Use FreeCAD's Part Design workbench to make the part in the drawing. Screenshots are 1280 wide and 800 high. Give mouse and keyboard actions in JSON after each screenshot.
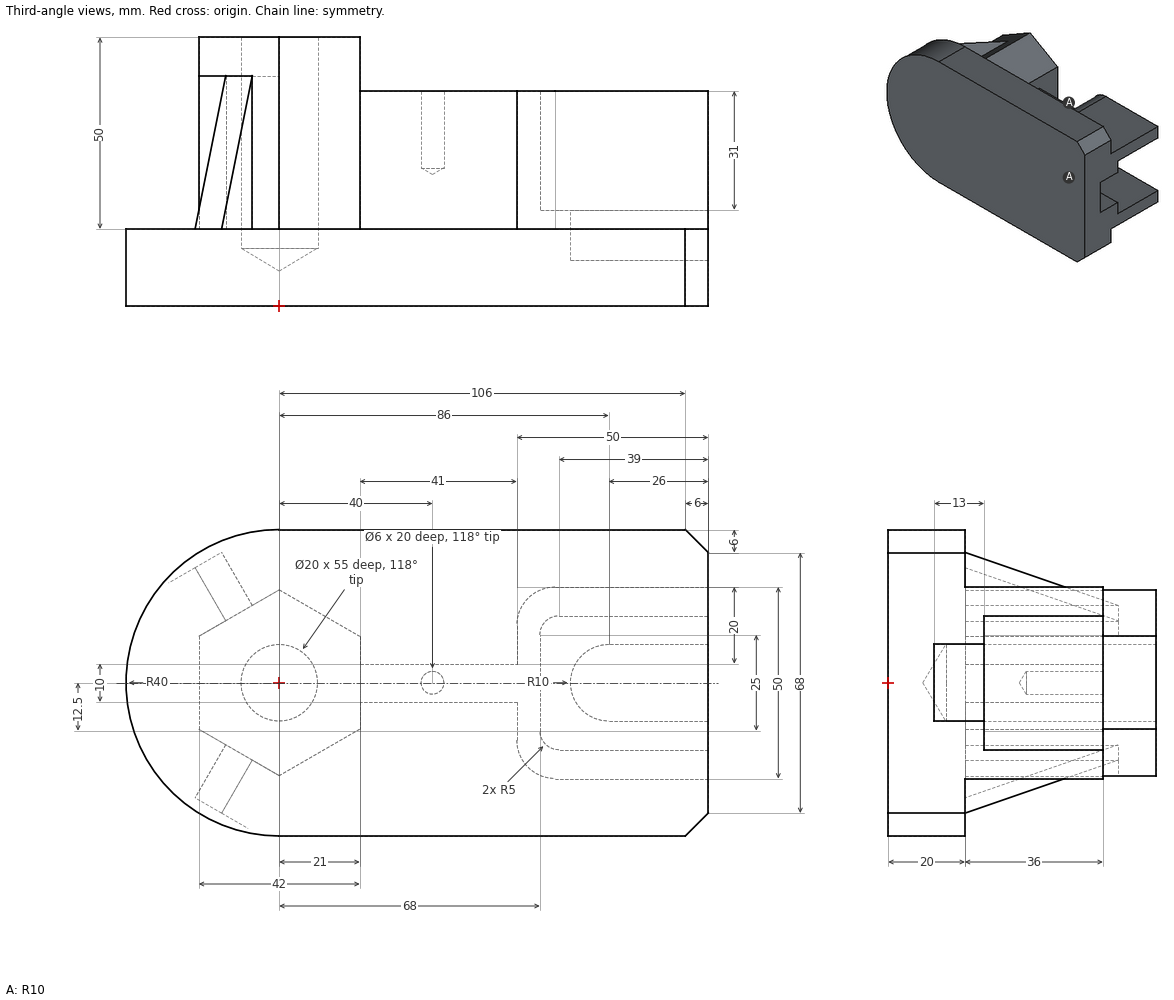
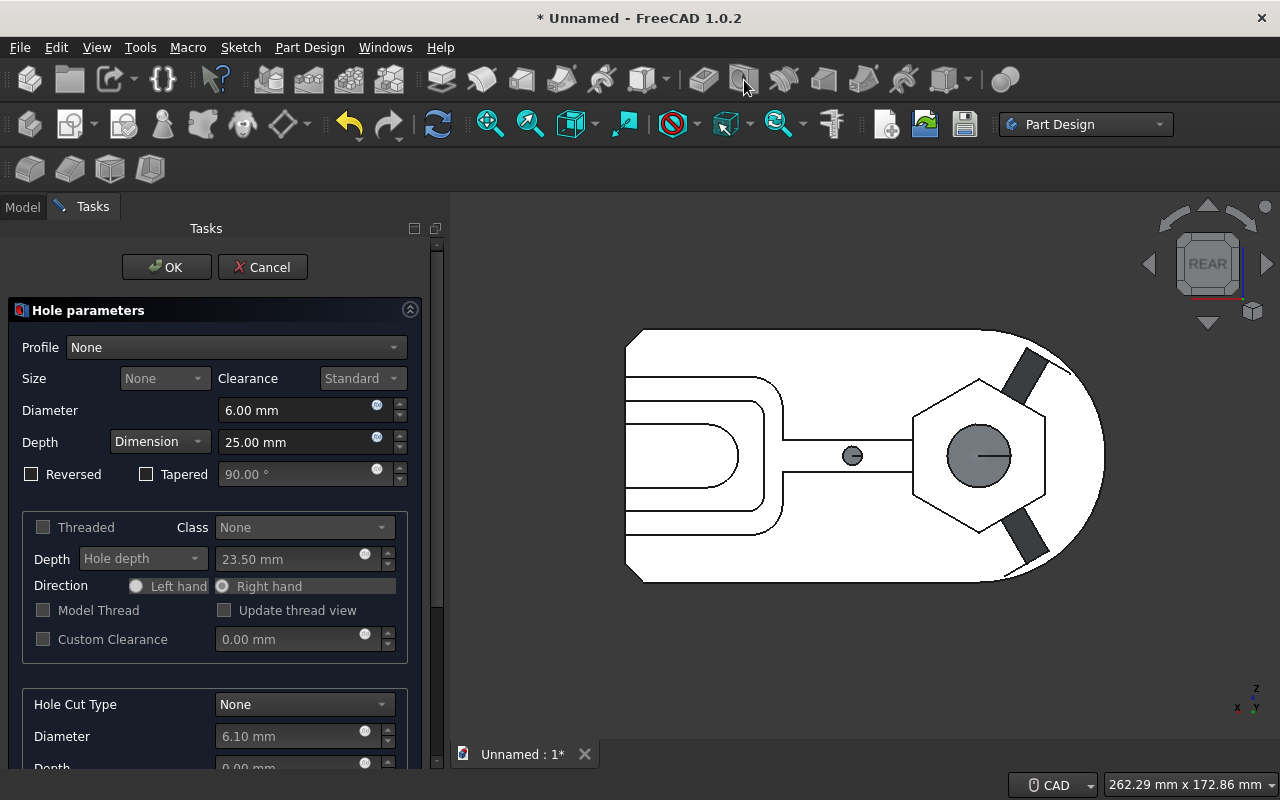
{"action": "triple_click", "coordinate": [305, 410]}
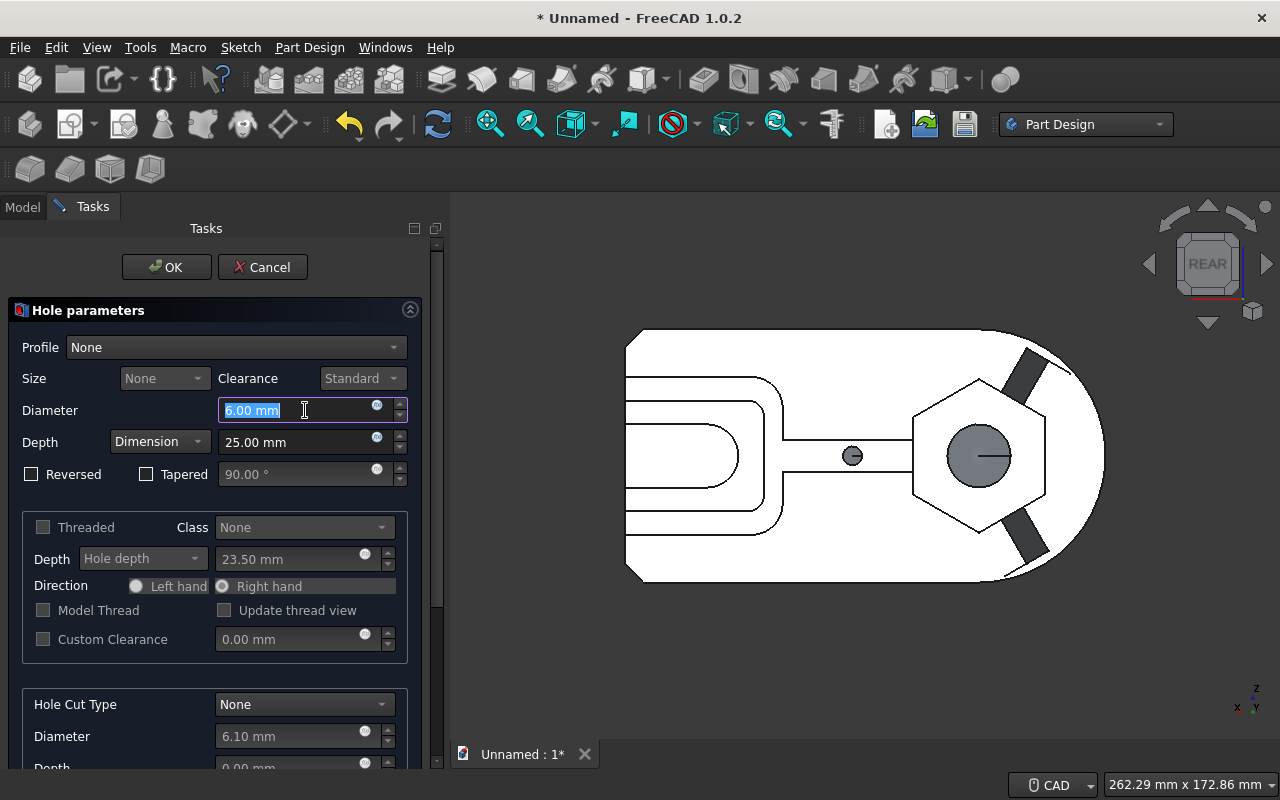
{"action": "type", "text": "6"}
{"action": "key", "text": "Tab"}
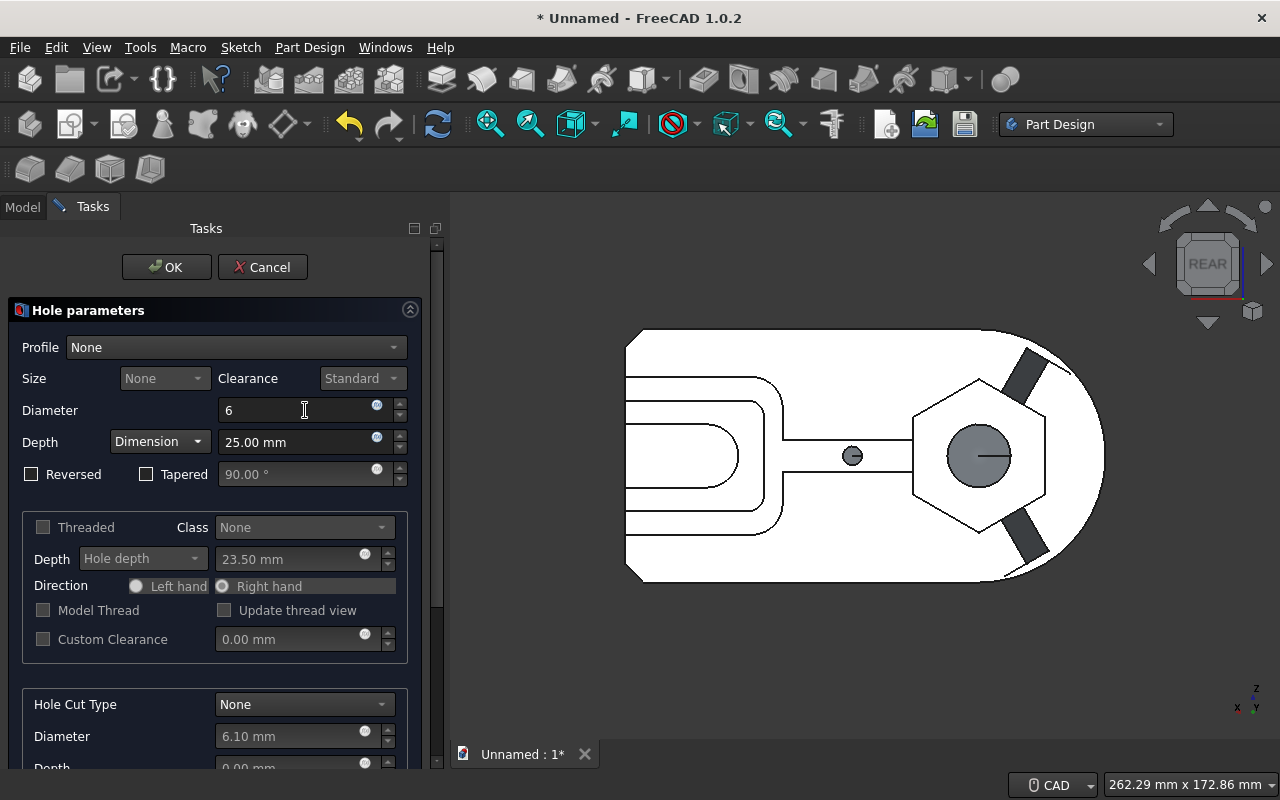
{"action": "triple_click", "coordinate": [305, 442]}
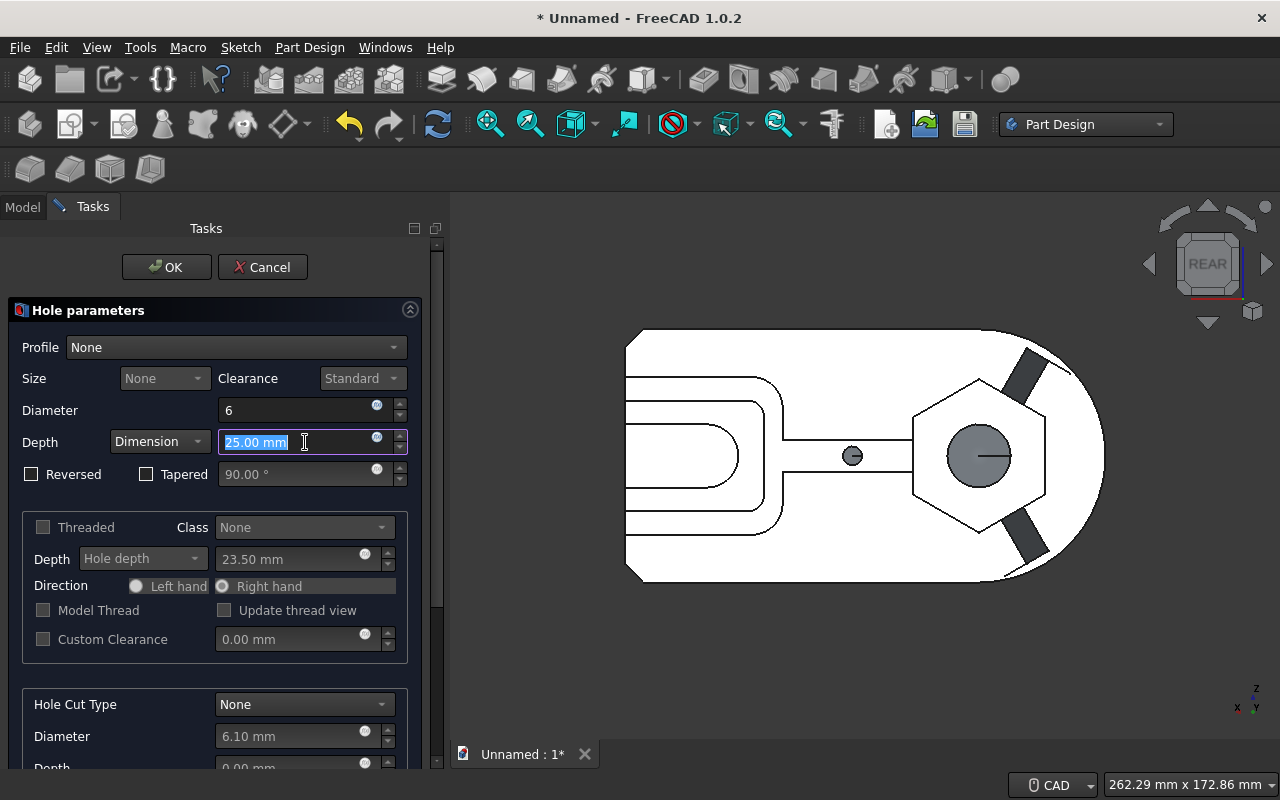
{"action": "type", "text": "20"}
{"action": "key", "text": "Tab"}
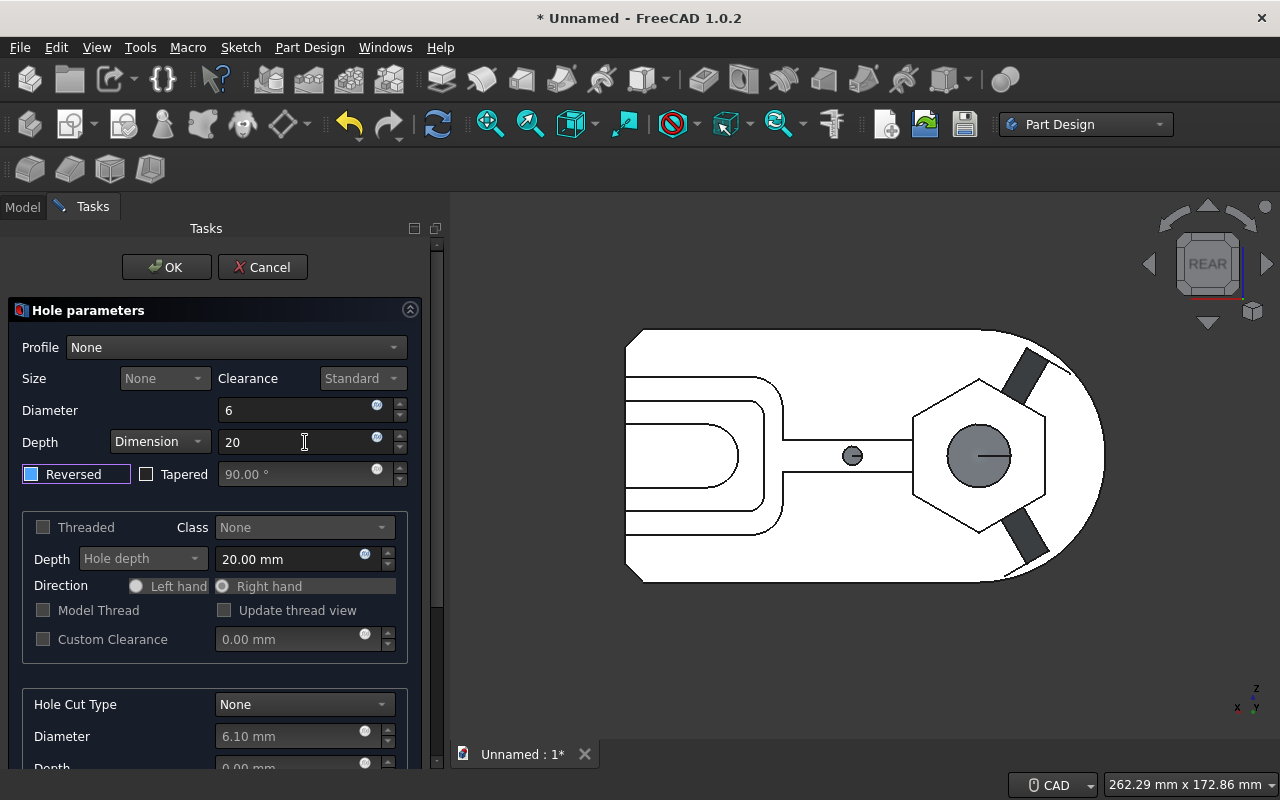
{"action": "left_click", "coordinate": [167, 267]}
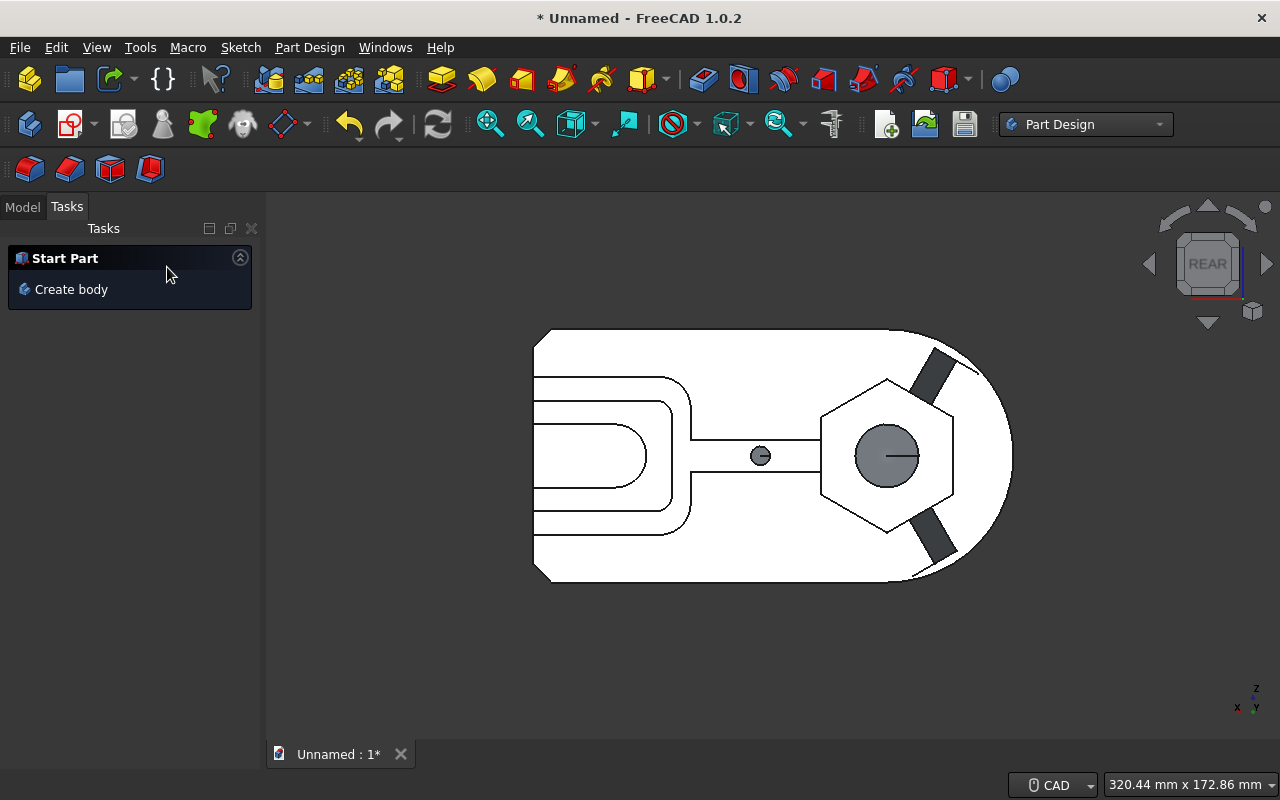
{"action": "key", "text": "0"}